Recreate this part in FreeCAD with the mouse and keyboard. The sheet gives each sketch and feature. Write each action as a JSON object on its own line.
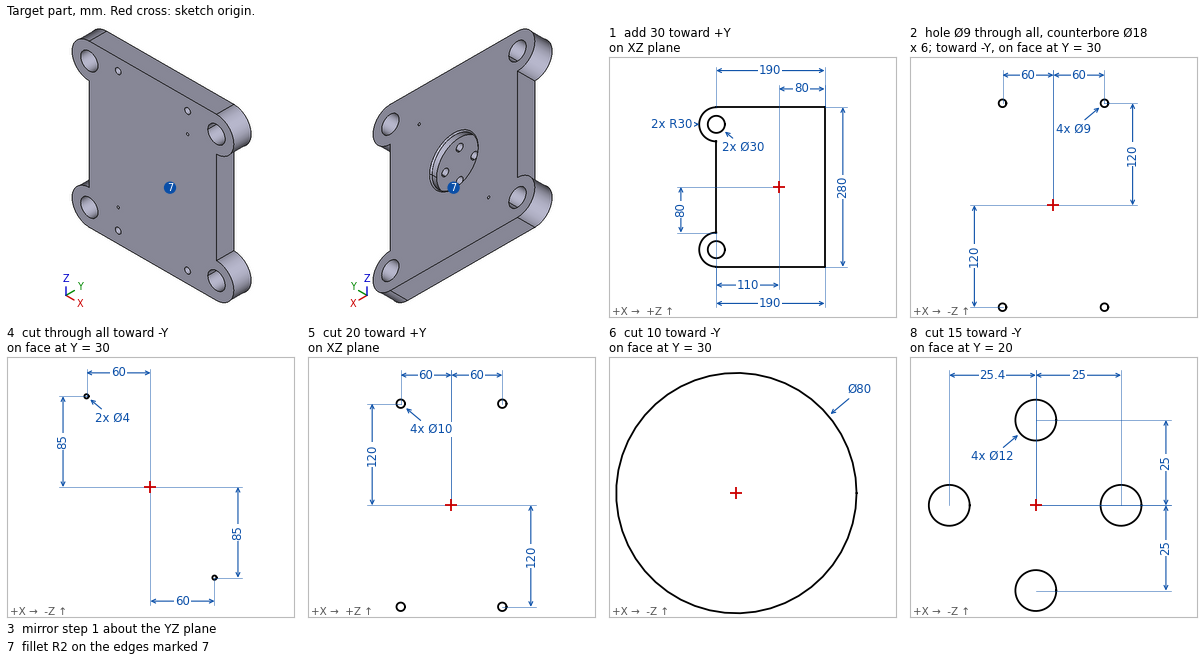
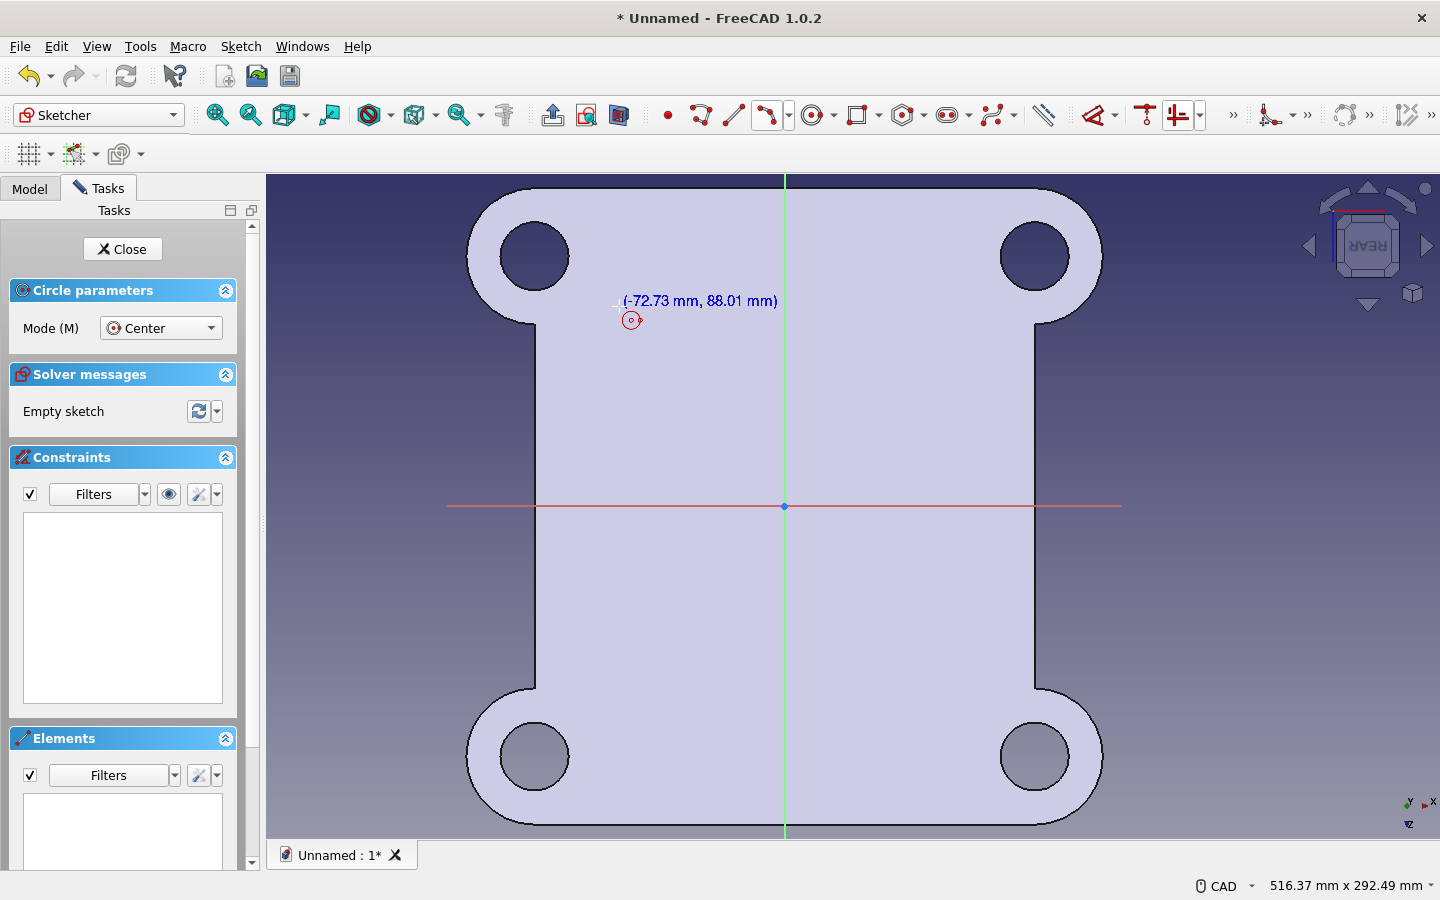
{"action": "left_click", "coordinate": [648, 313]}
{"action": "mouse_move", "coordinate": [651, 310]}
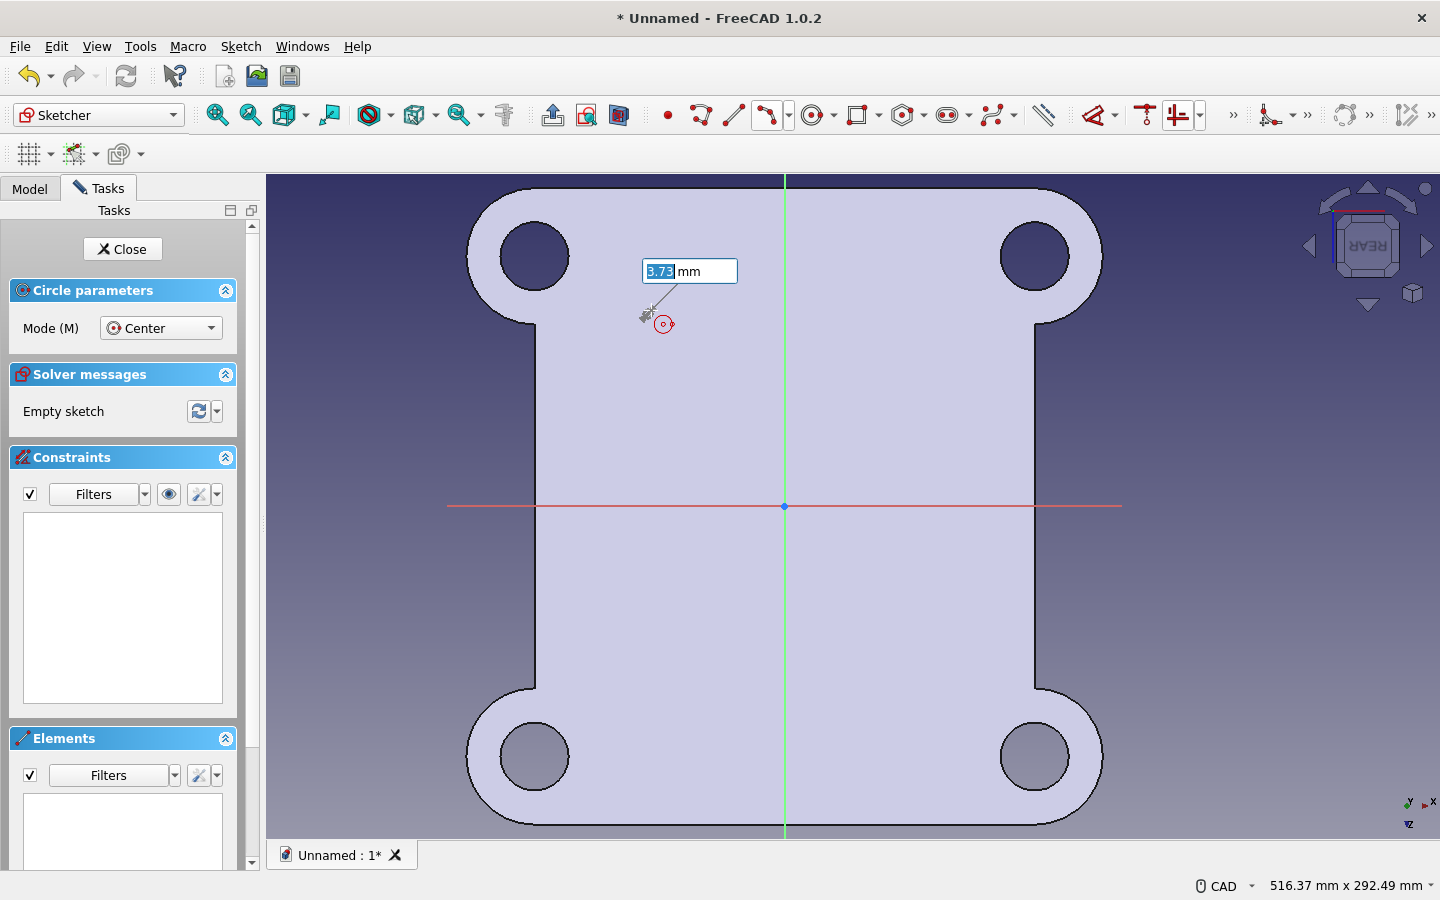
{"action": "type", "text": "4"}
{"action": "key", "text": "Return"}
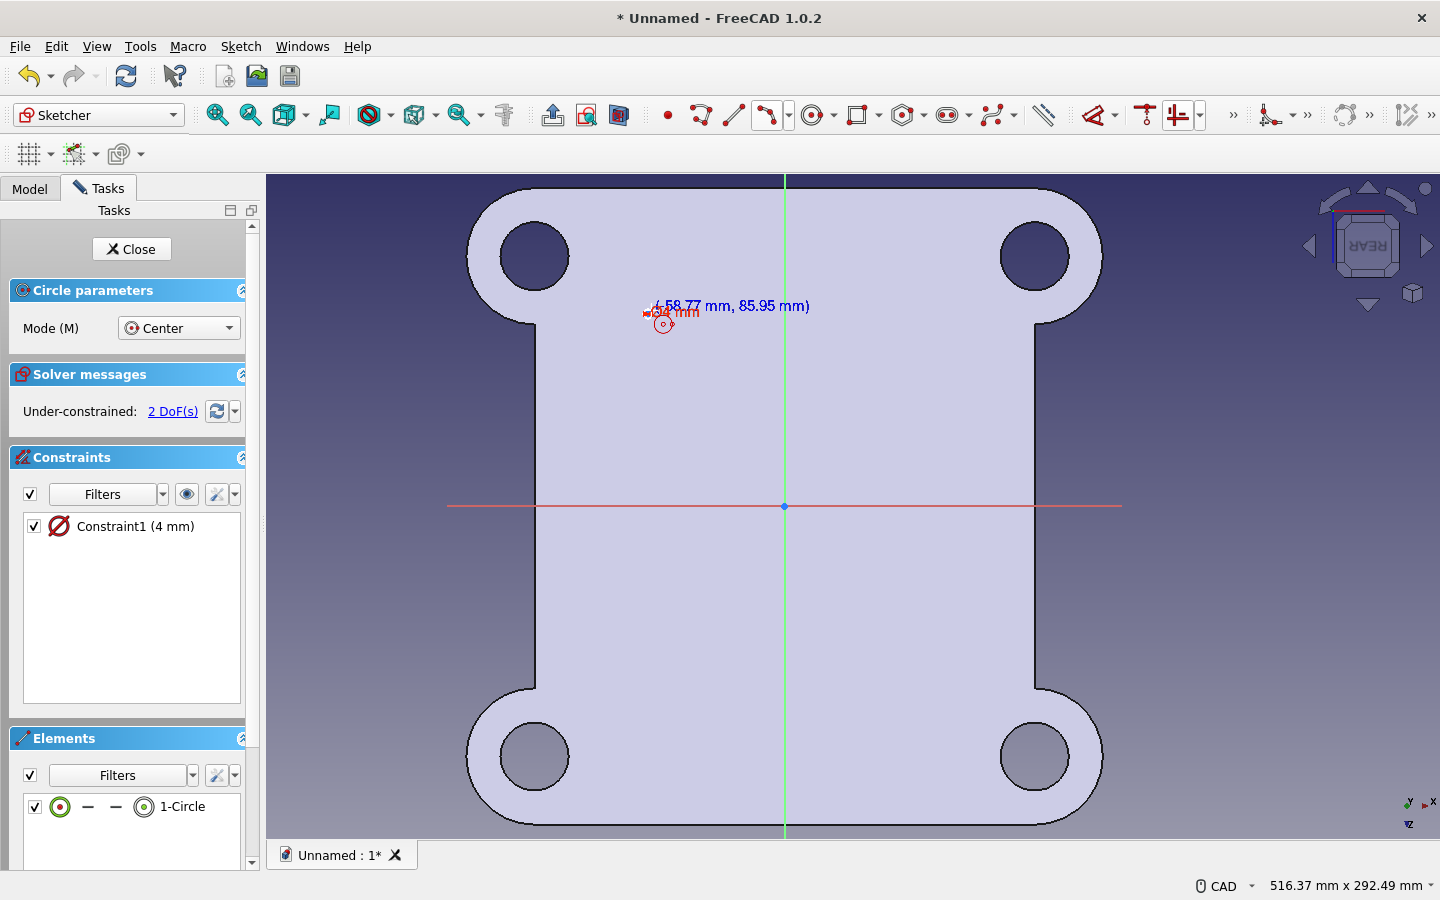
{"action": "scroll", "coordinate": [921, 700], "scroll_direction": "up", "scroll_amount": 9}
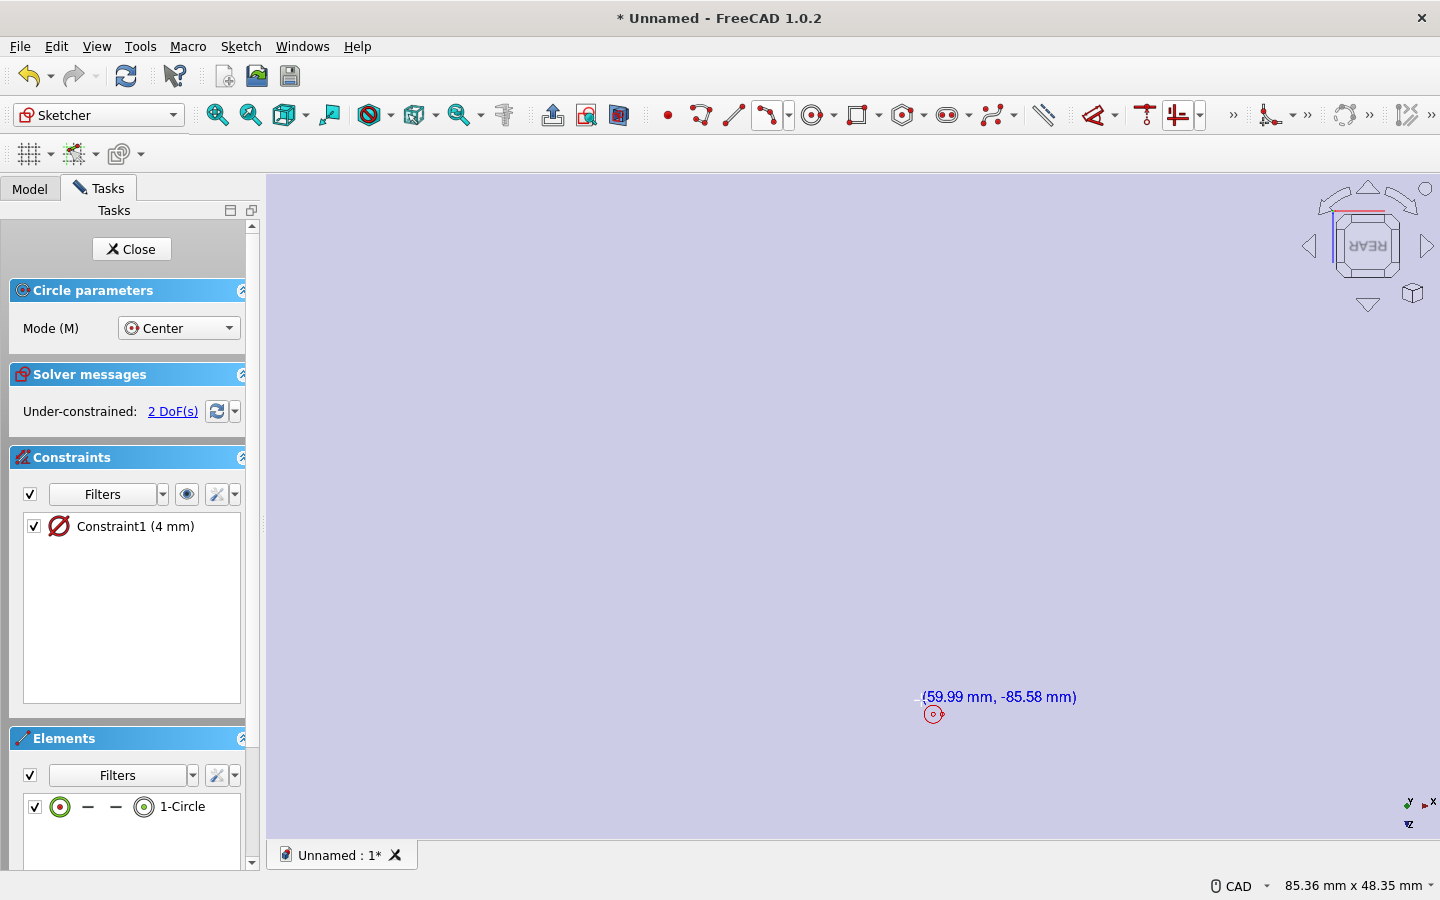
{"action": "scroll", "coordinate": [921, 701], "scroll_direction": "down", "scroll_amount": 9}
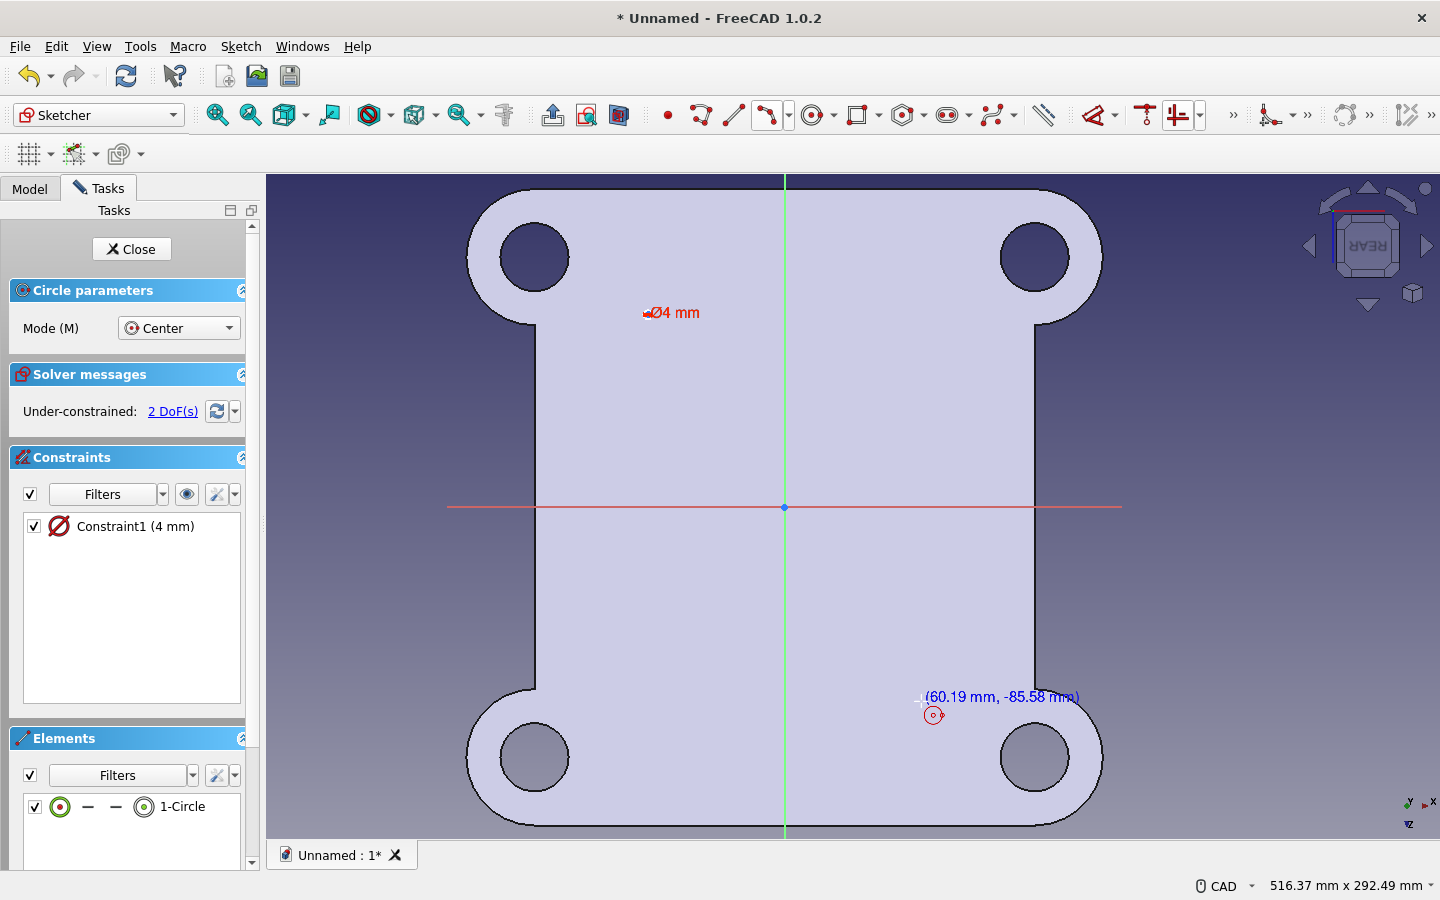
{"action": "left_click", "coordinate": [921, 701]}
{"action": "mouse_move", "coordinate": [924, 697]}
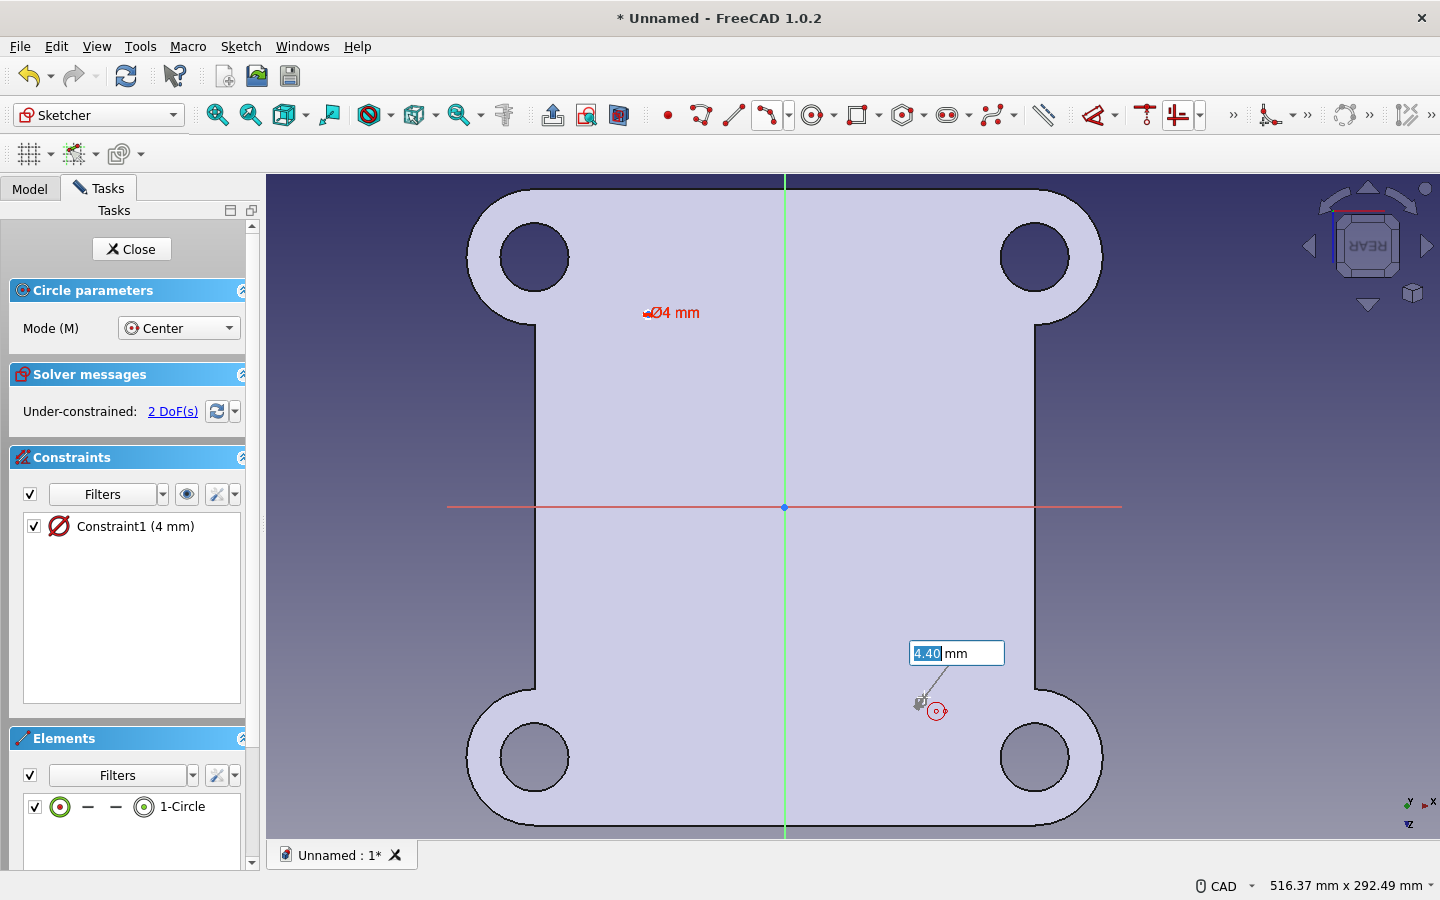
{"action": "type", "text": "4"}
{"action": "key", "text": "Return"}
{"action": "key", "text": "Escape"}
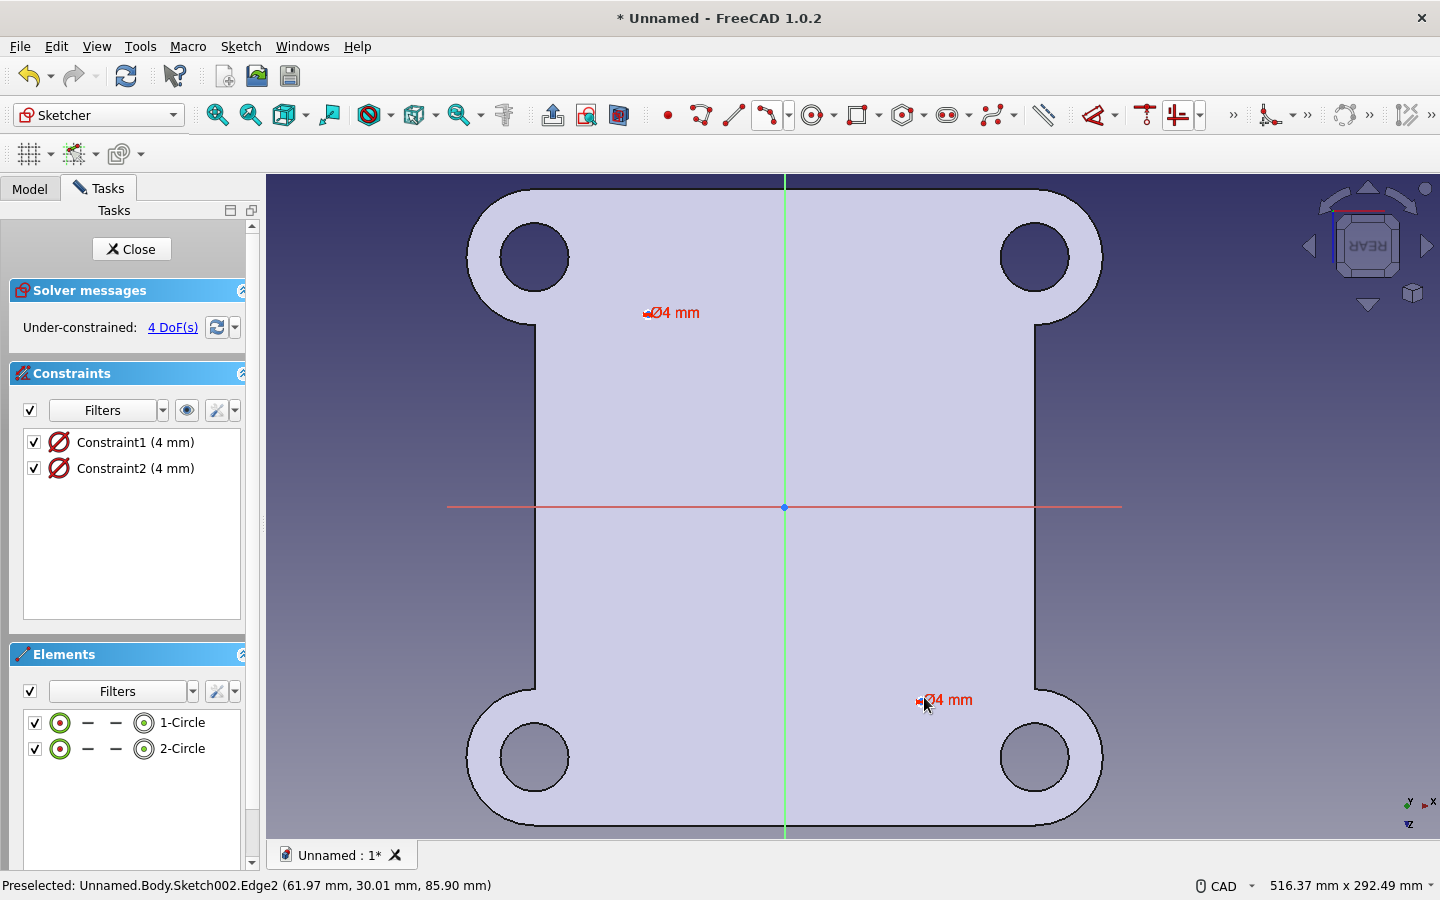
{"action": "key", "text": "d"}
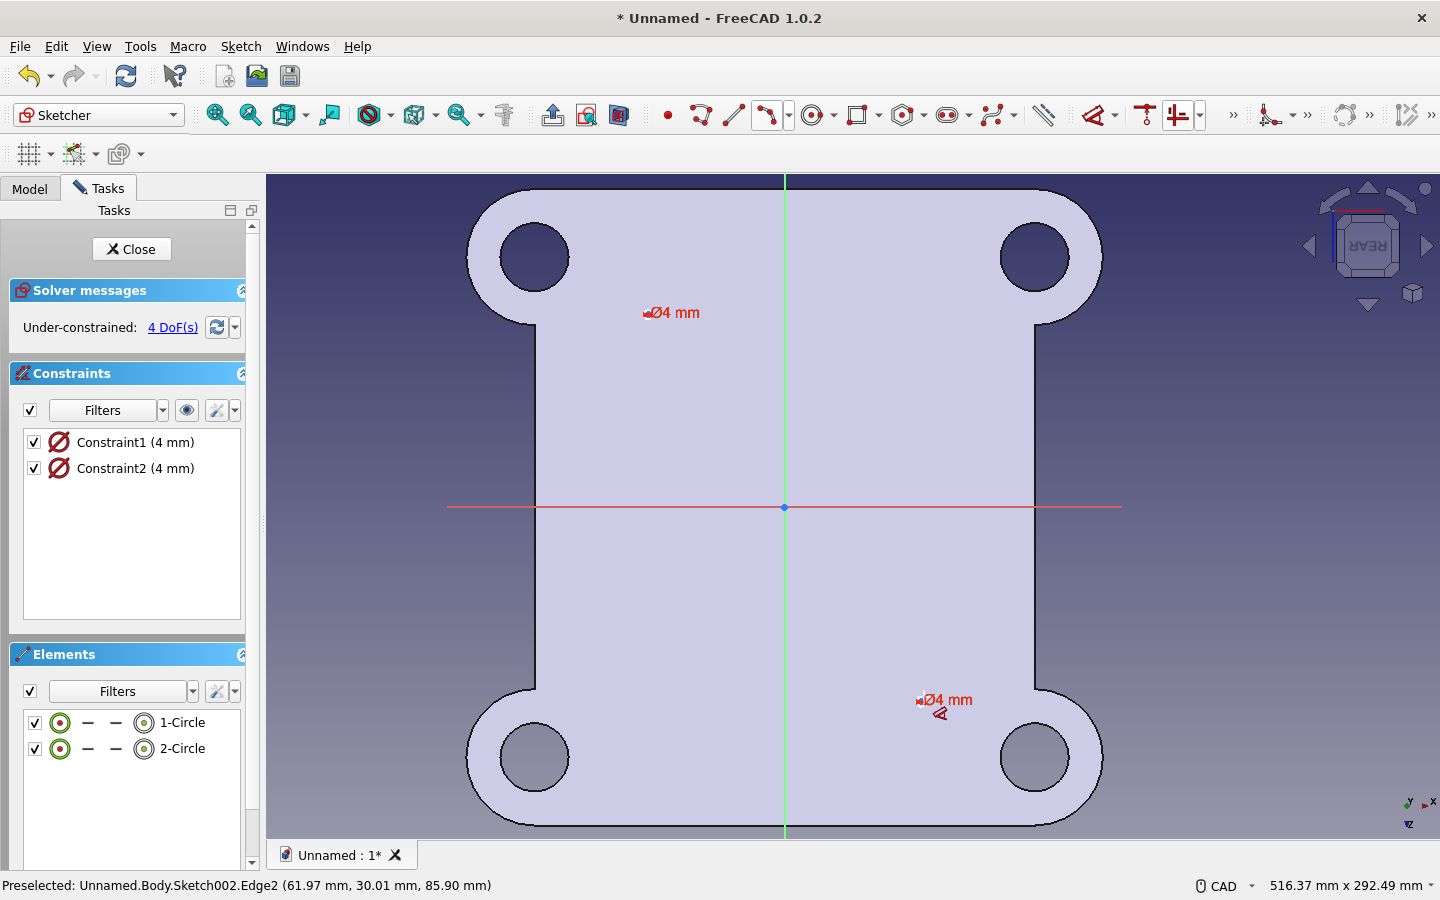
{"action": "left_click", "coordinate": [648, 315]}
{"action": "left_click", "coordinate": [716, 281]}